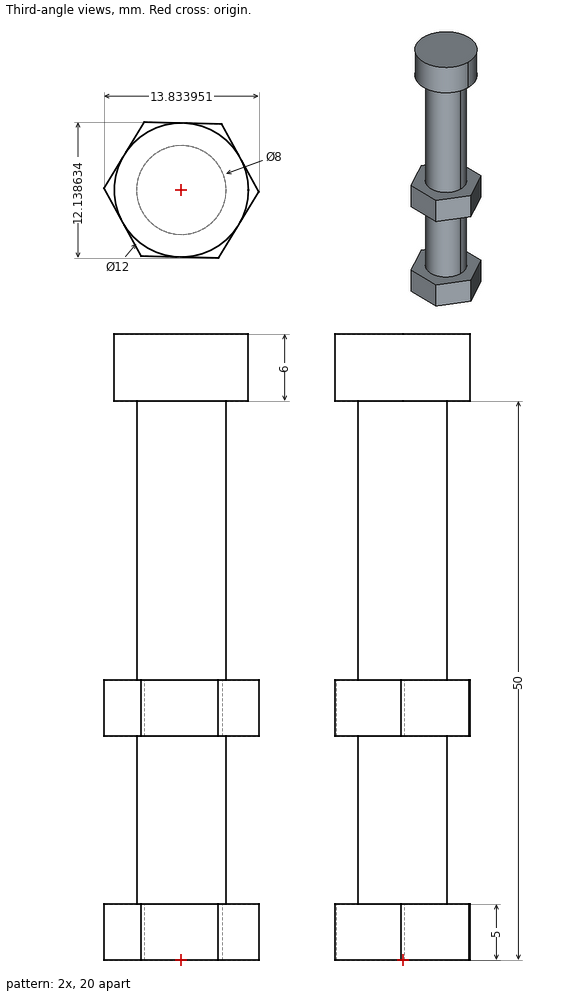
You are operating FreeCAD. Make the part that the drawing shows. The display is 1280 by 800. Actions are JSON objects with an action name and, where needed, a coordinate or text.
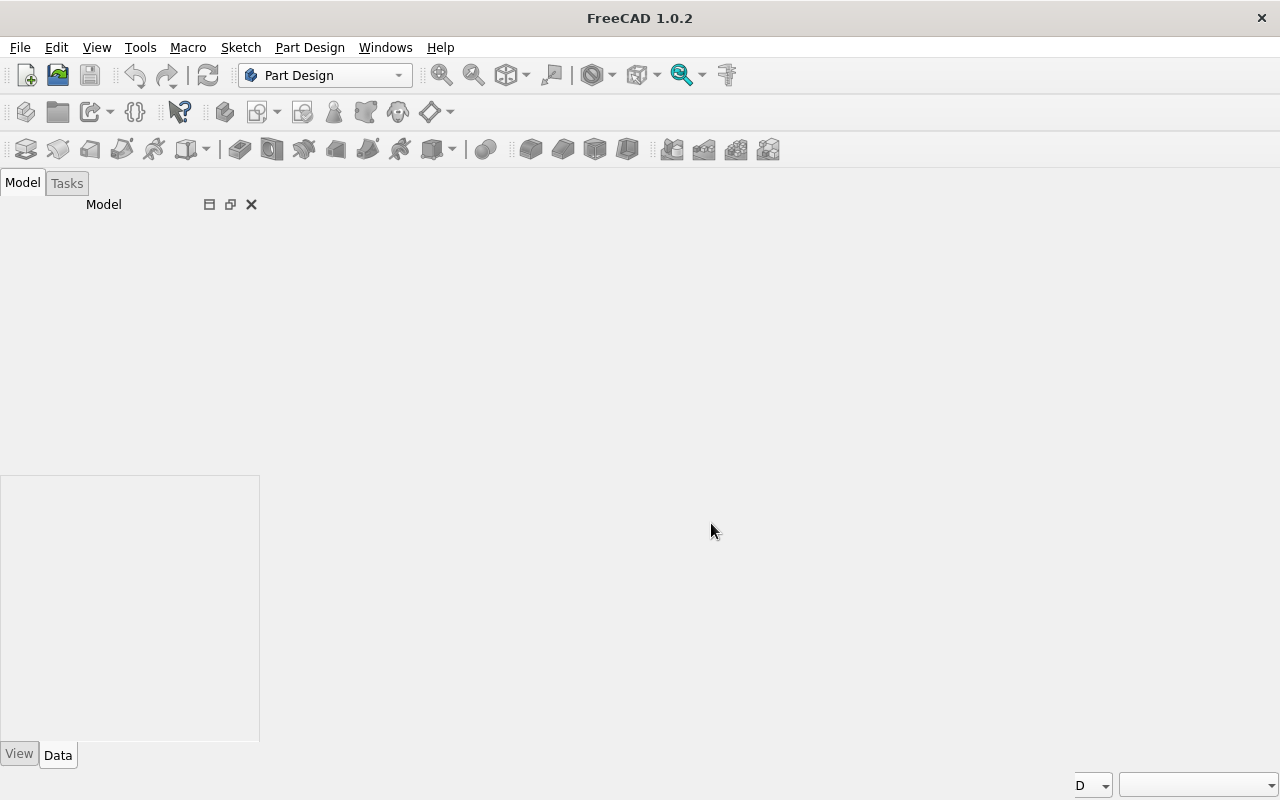
{"action": "left_click", "coordinate": [26, 76]}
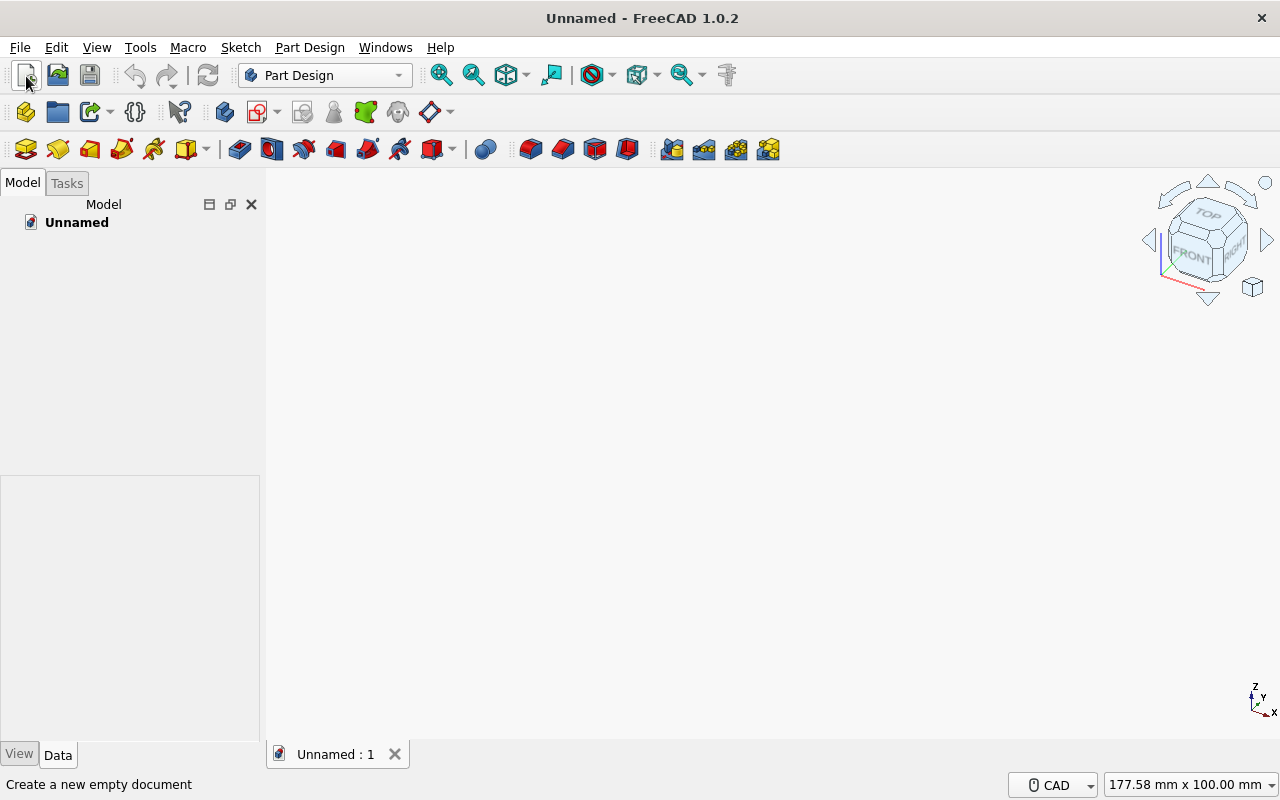
{"action": "left_click", "coordinate": [258, 112]}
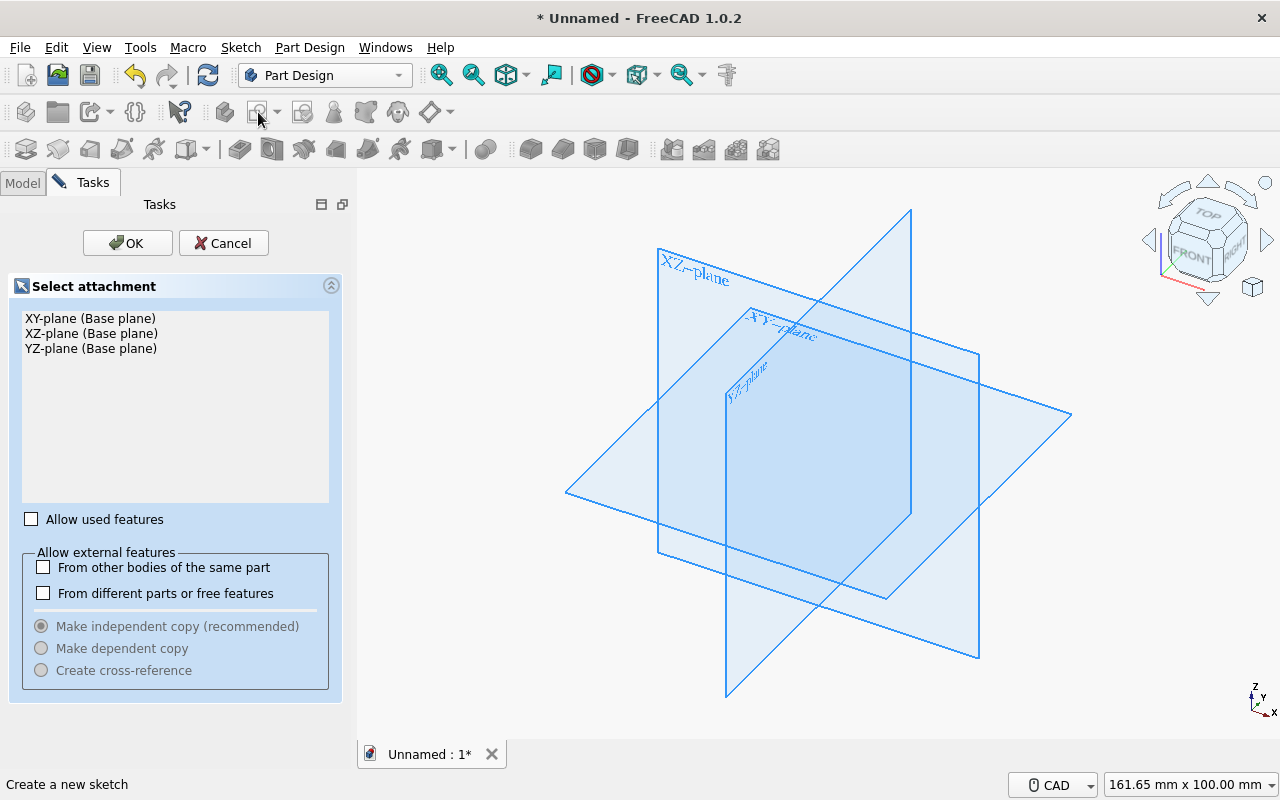
{"action": "left_click", "coordinate": [82, 318]}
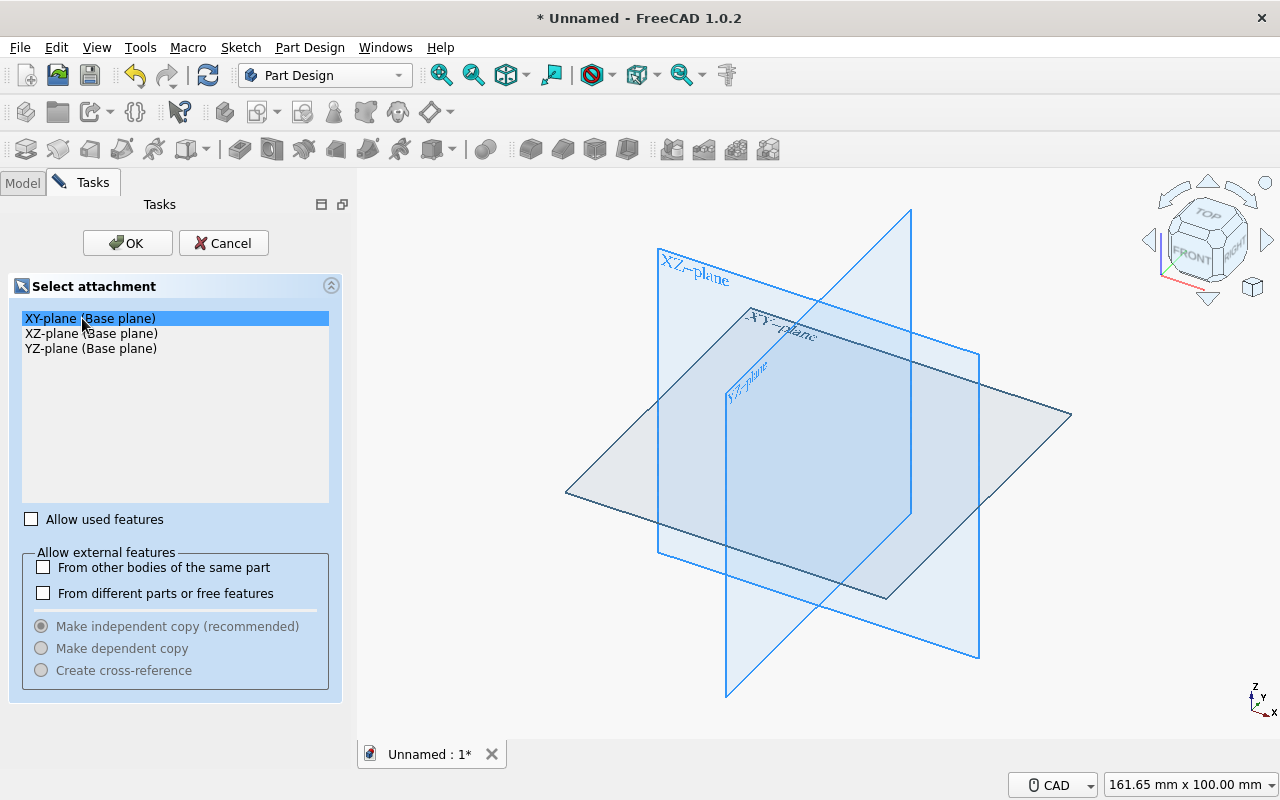
{"action": "left_click", "coordinate": [128, 243]}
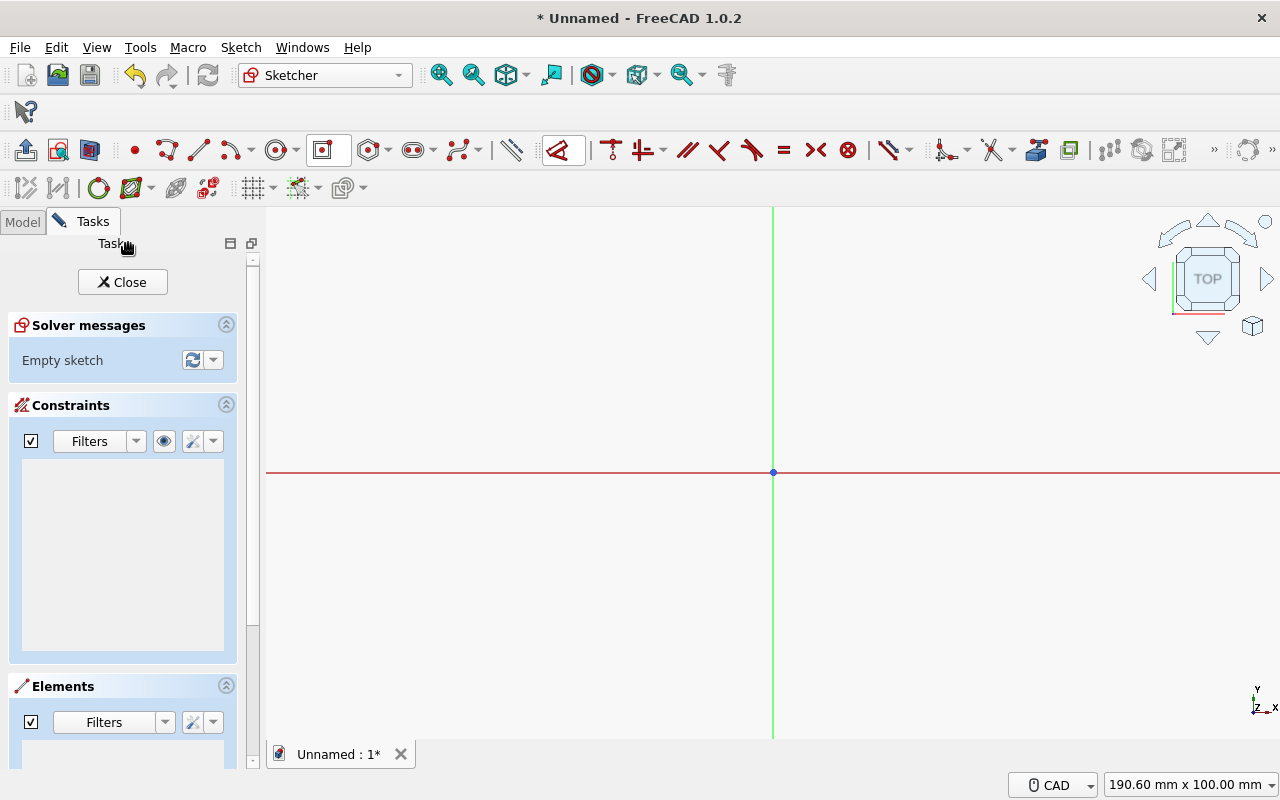
{"action": "scroll", "coordinate": [784, 473], "scroll_direction": "up", "scroll_amount": 10}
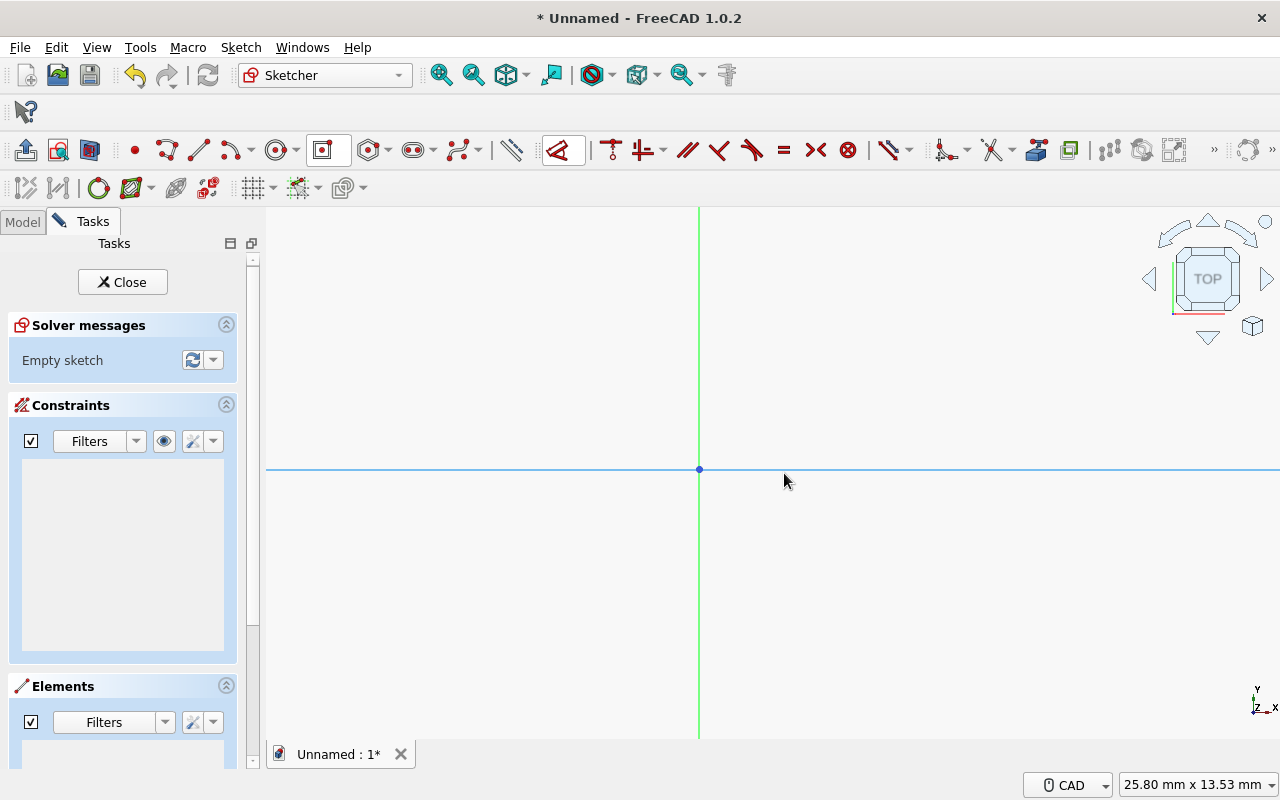
{"action": "left_click", "coordinate": [276, 150]}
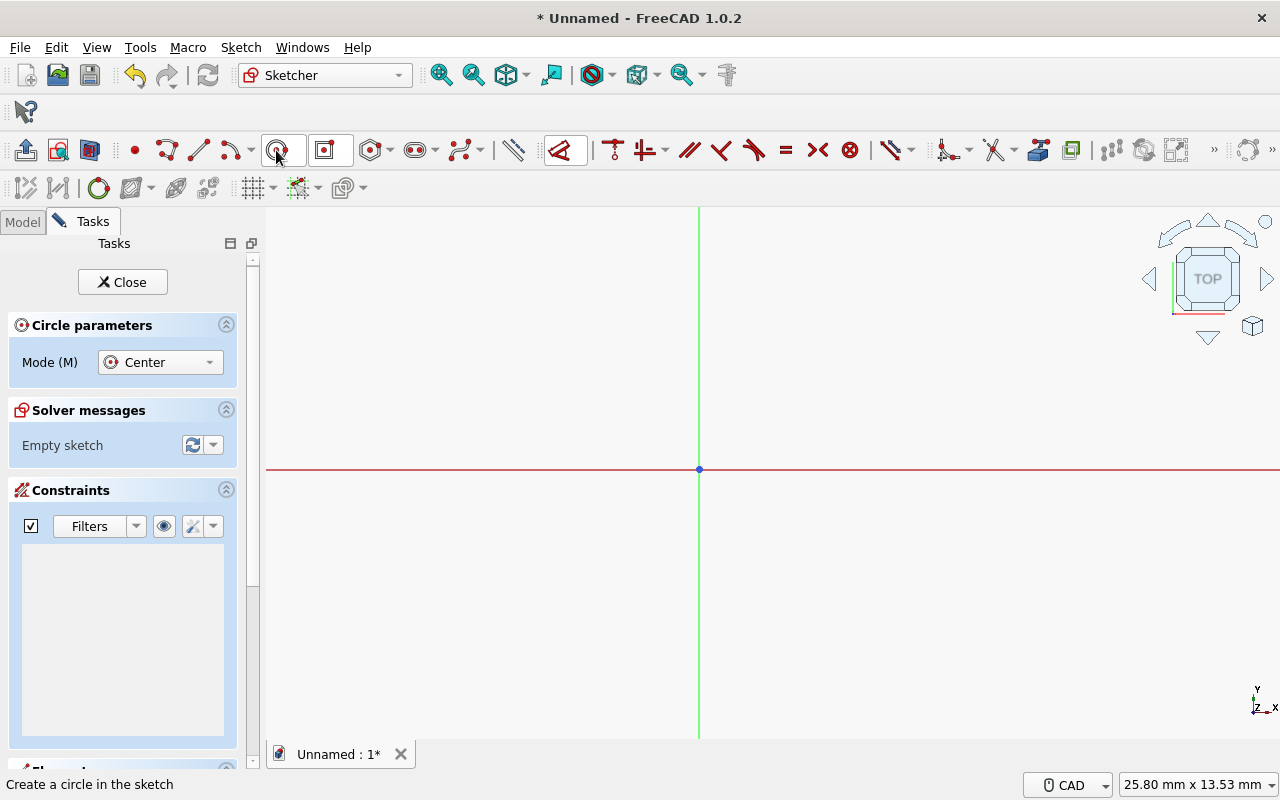
{"action": "left_click", "coordinate": [699, 470]}
{"action": "mouse_move", "coordinate": [811, 359]}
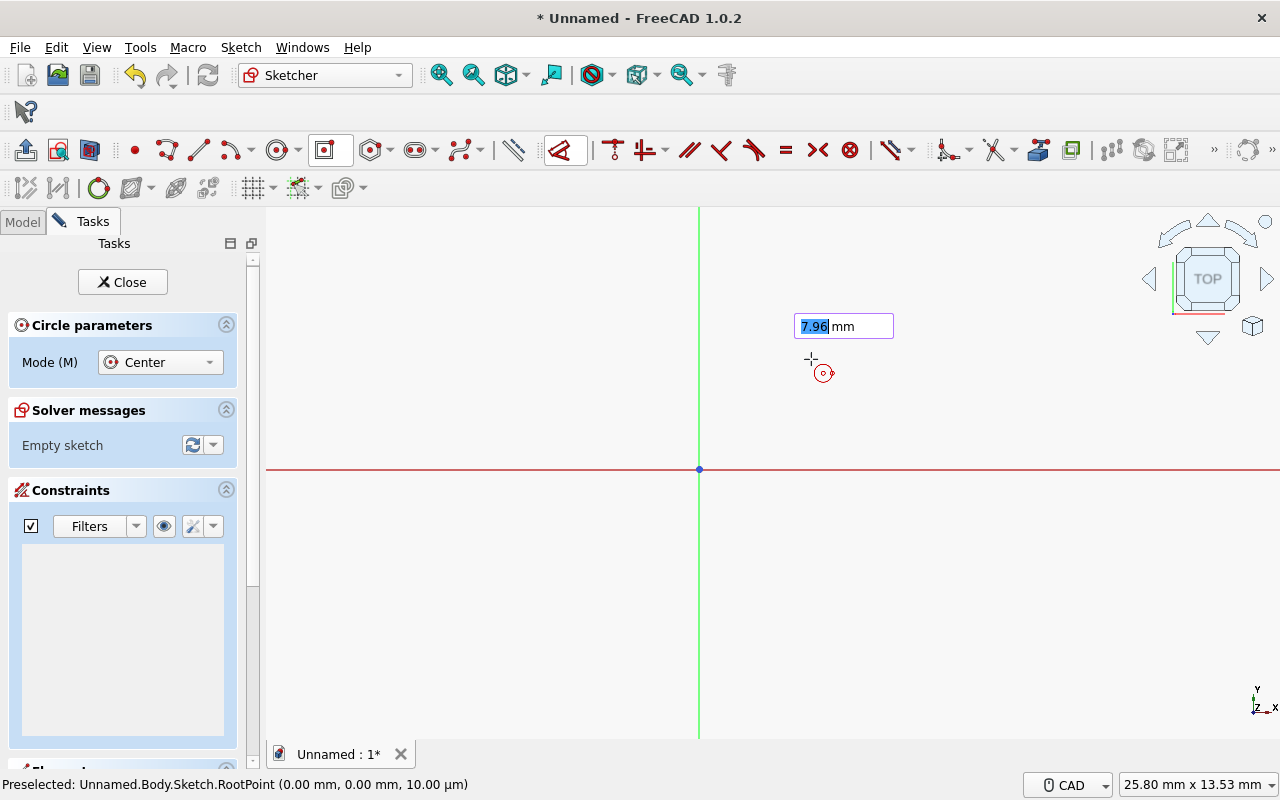
{"action": "type", "text": "8"}
{"action": "key", "text": "Return"}
{"action": "key", "text": "Escape"}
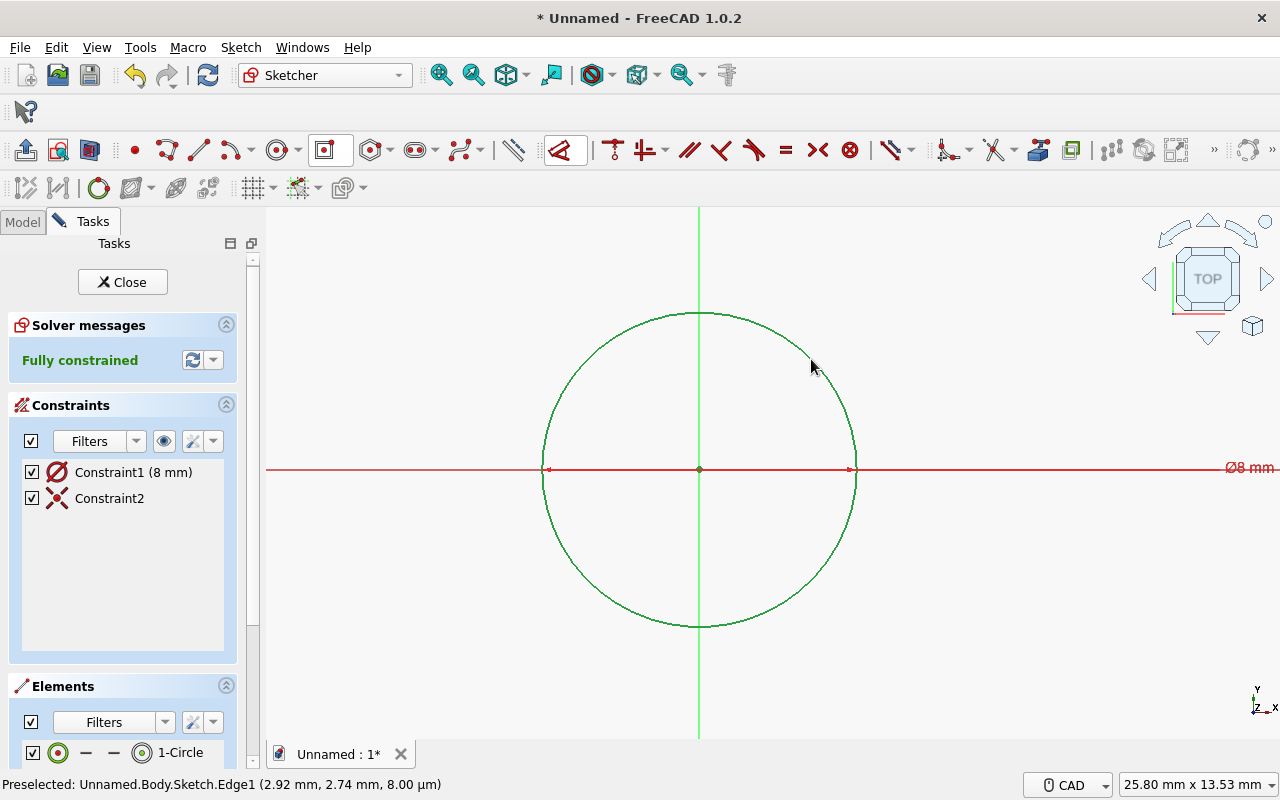
{"action": "left_click", "coordinate": [123, 282]}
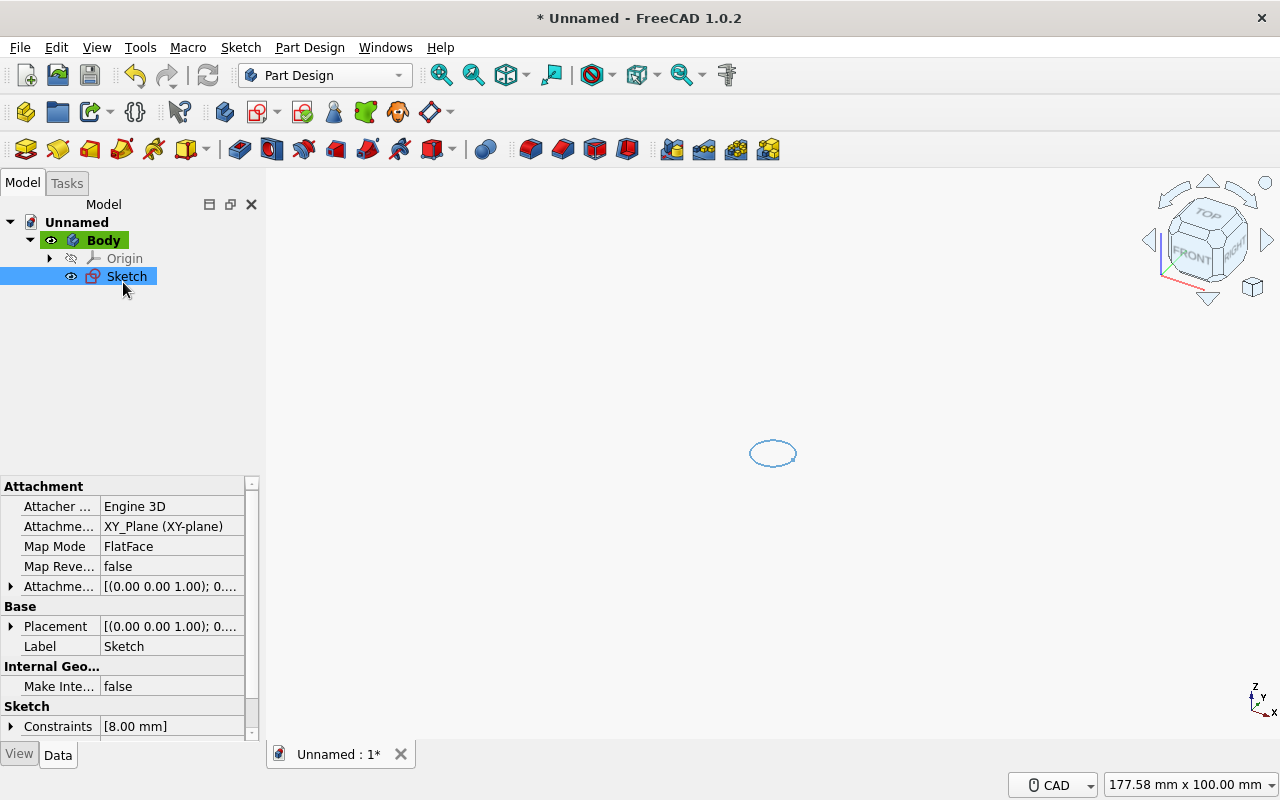
{"action": "left_click", "coordinate": [26, 150]}